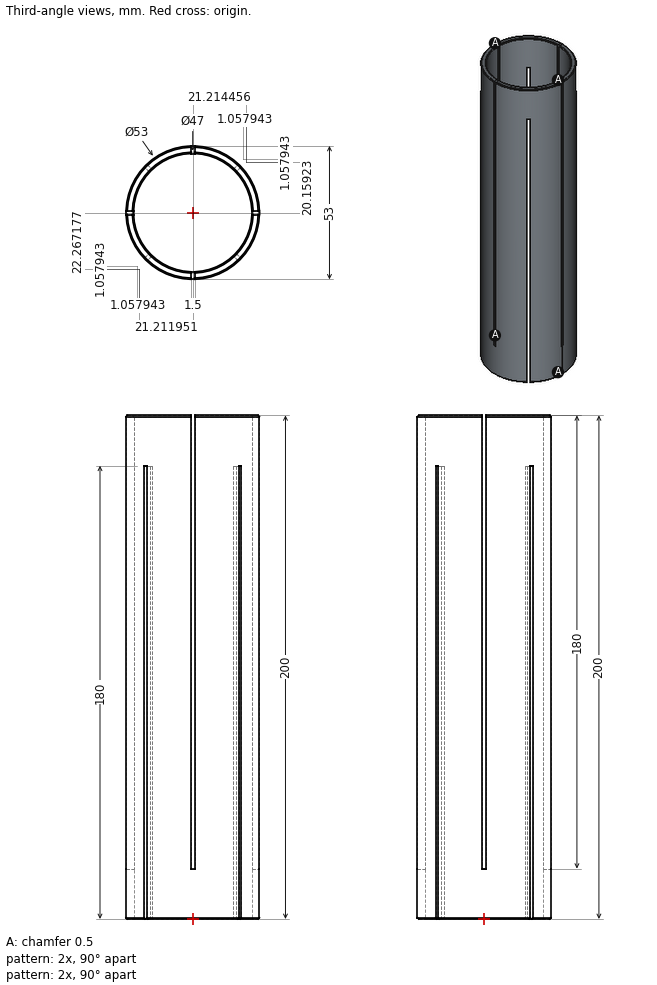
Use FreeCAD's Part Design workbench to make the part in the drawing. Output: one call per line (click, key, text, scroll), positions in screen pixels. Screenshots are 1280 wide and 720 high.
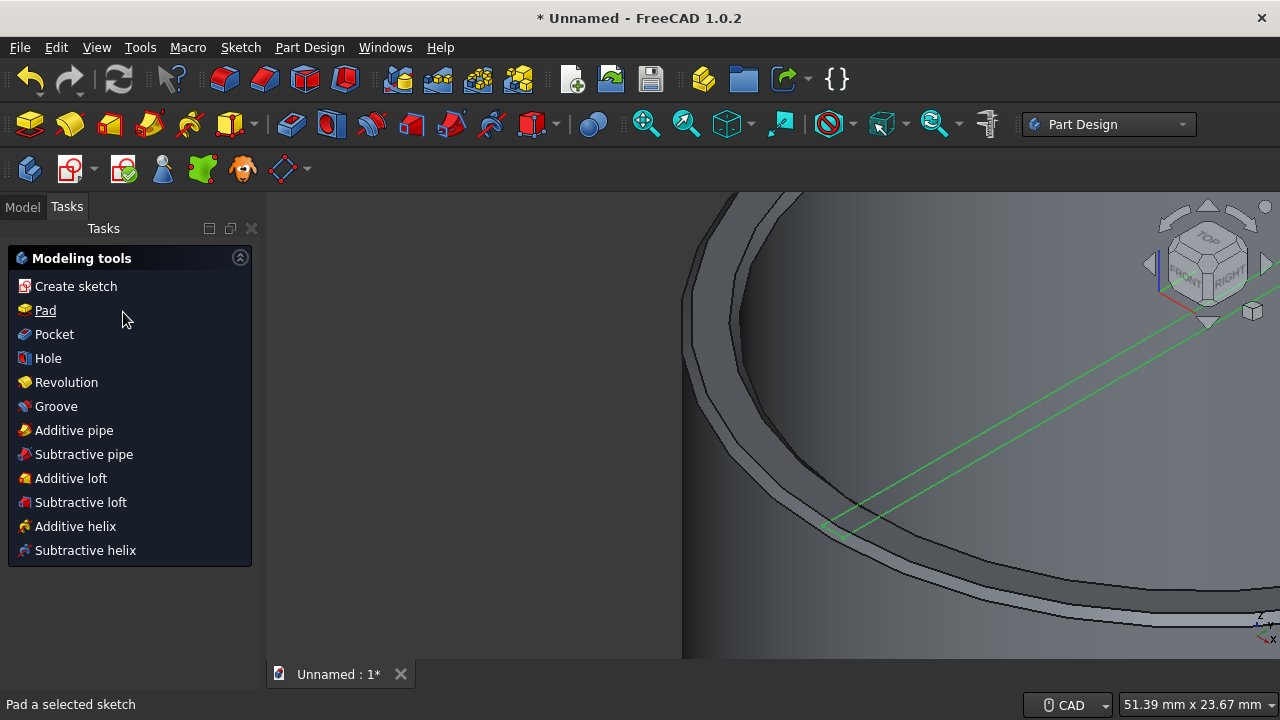
click(292, 124)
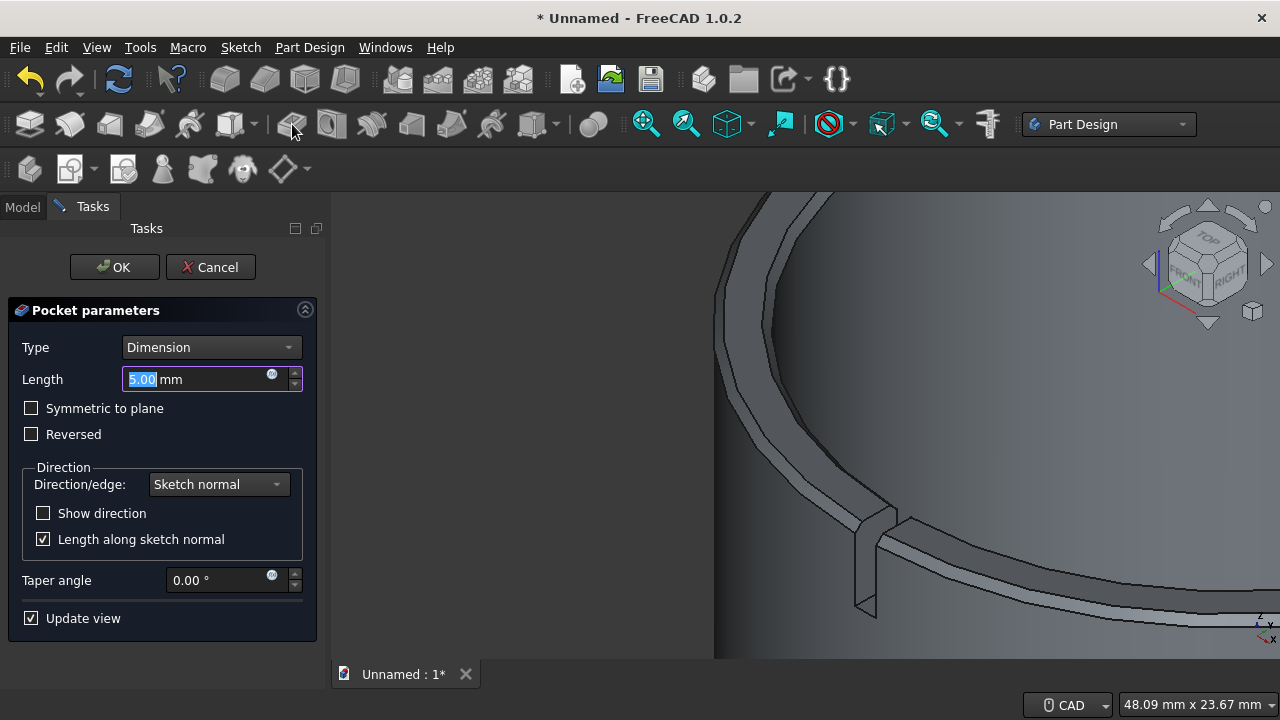
text(180)
key(Tab)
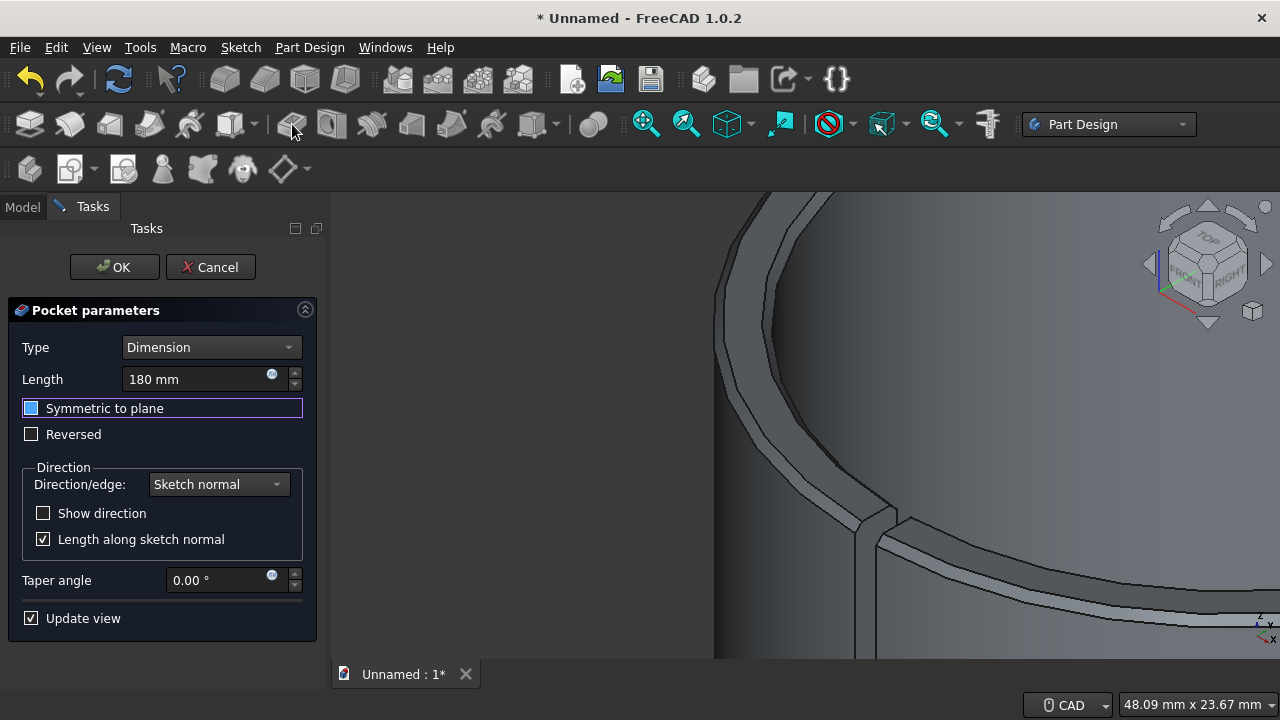
click(115, 267)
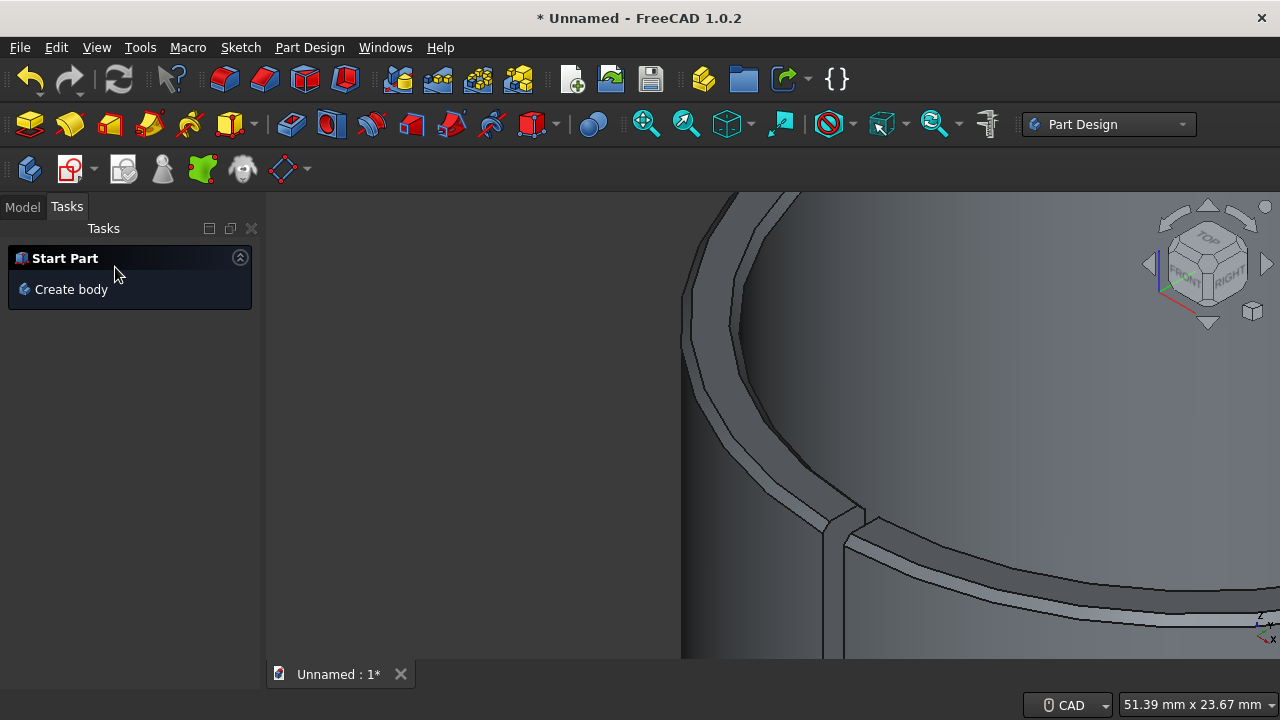
click(648, 124)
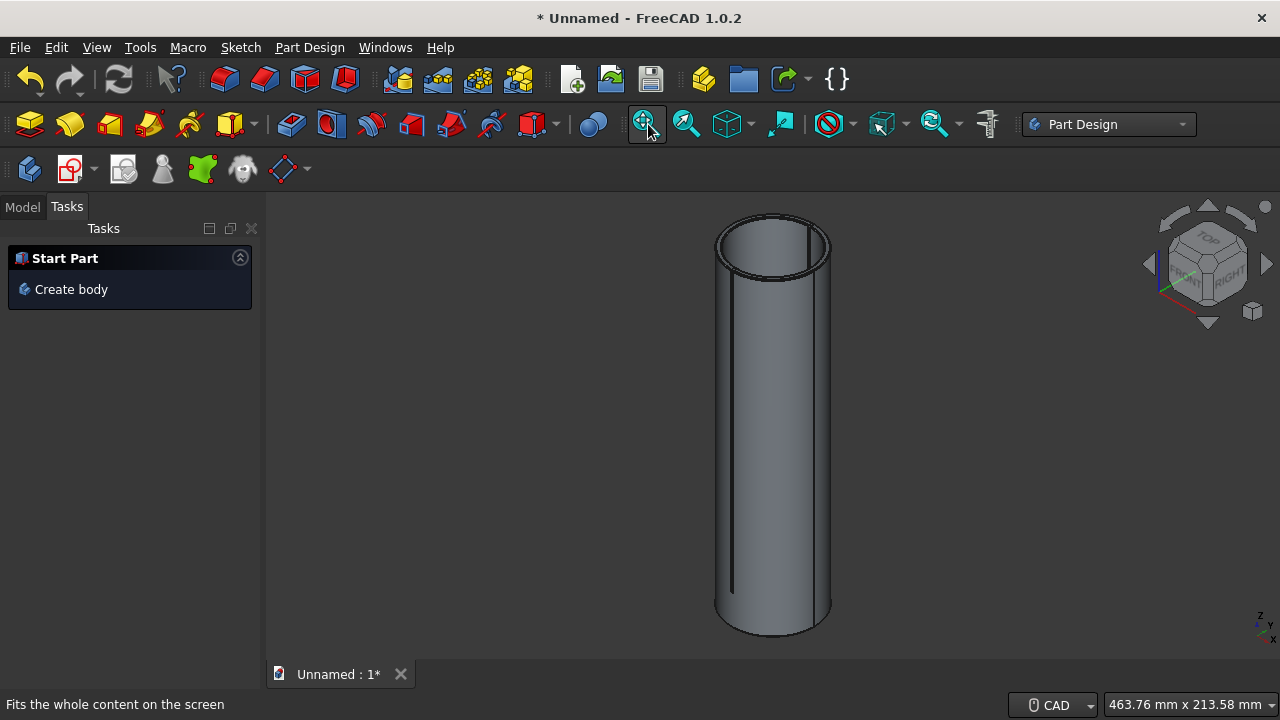
click(23, 206)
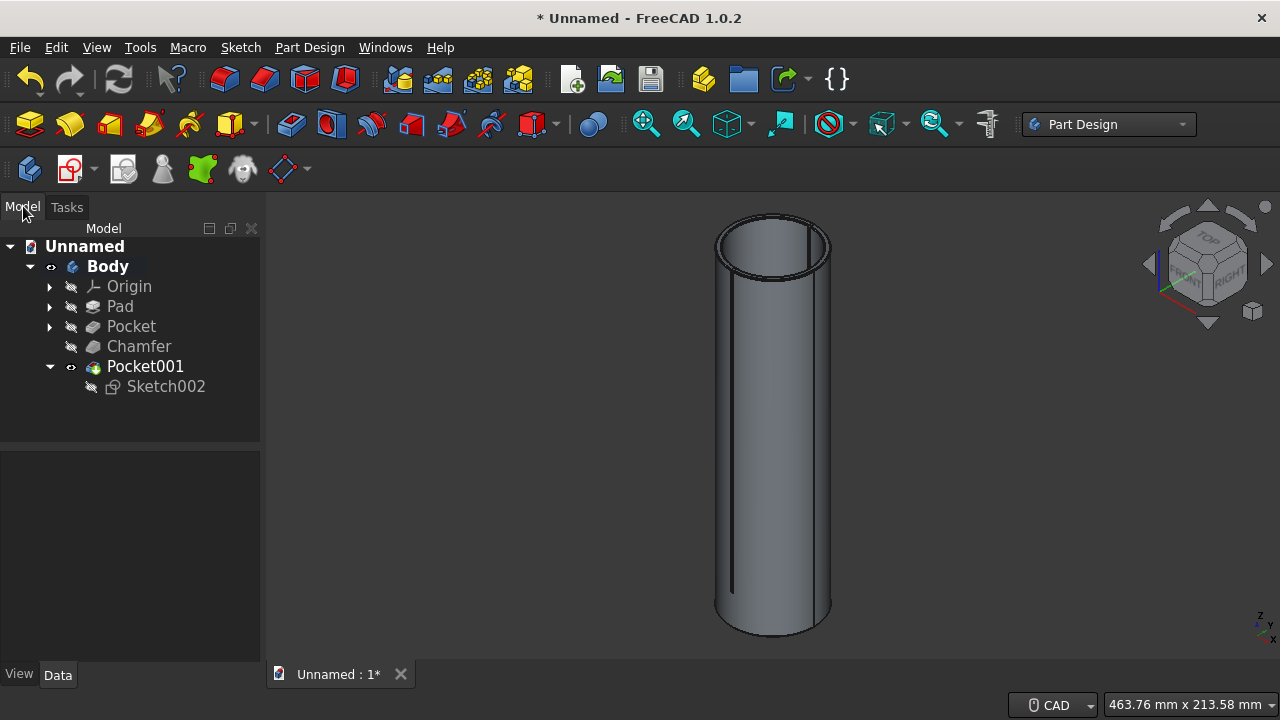
click(116, 367)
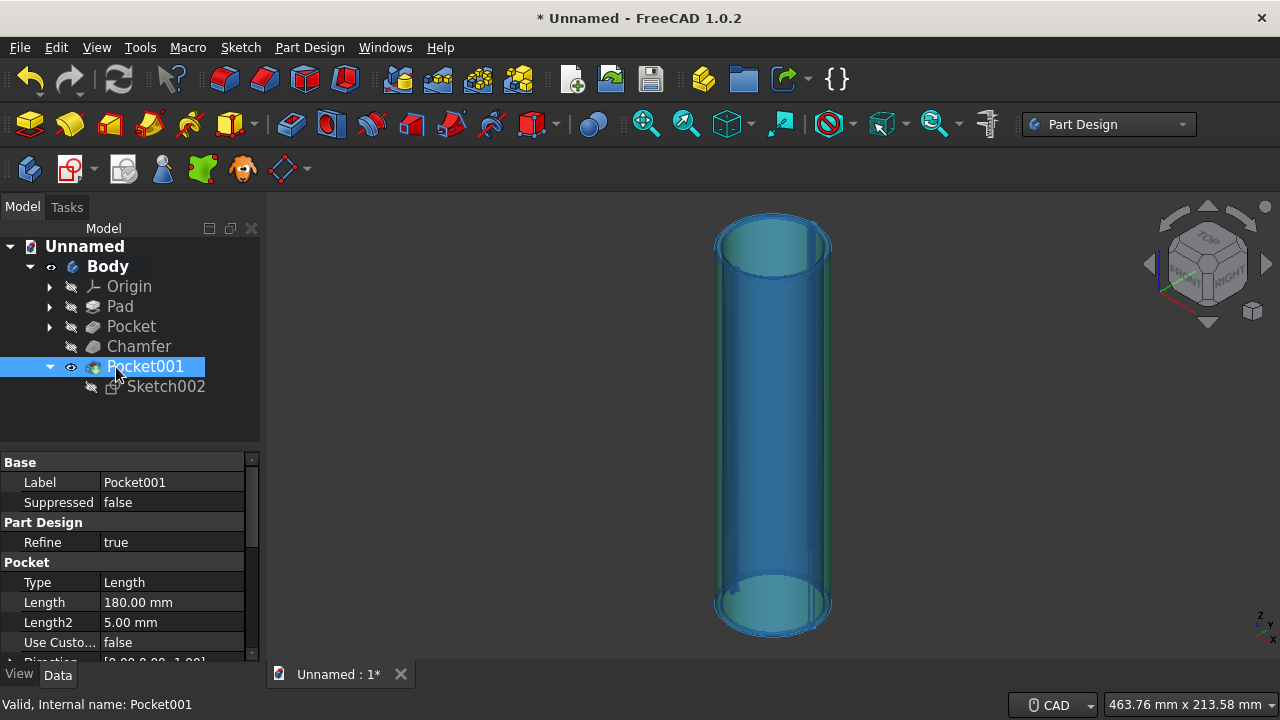
click(478, 80)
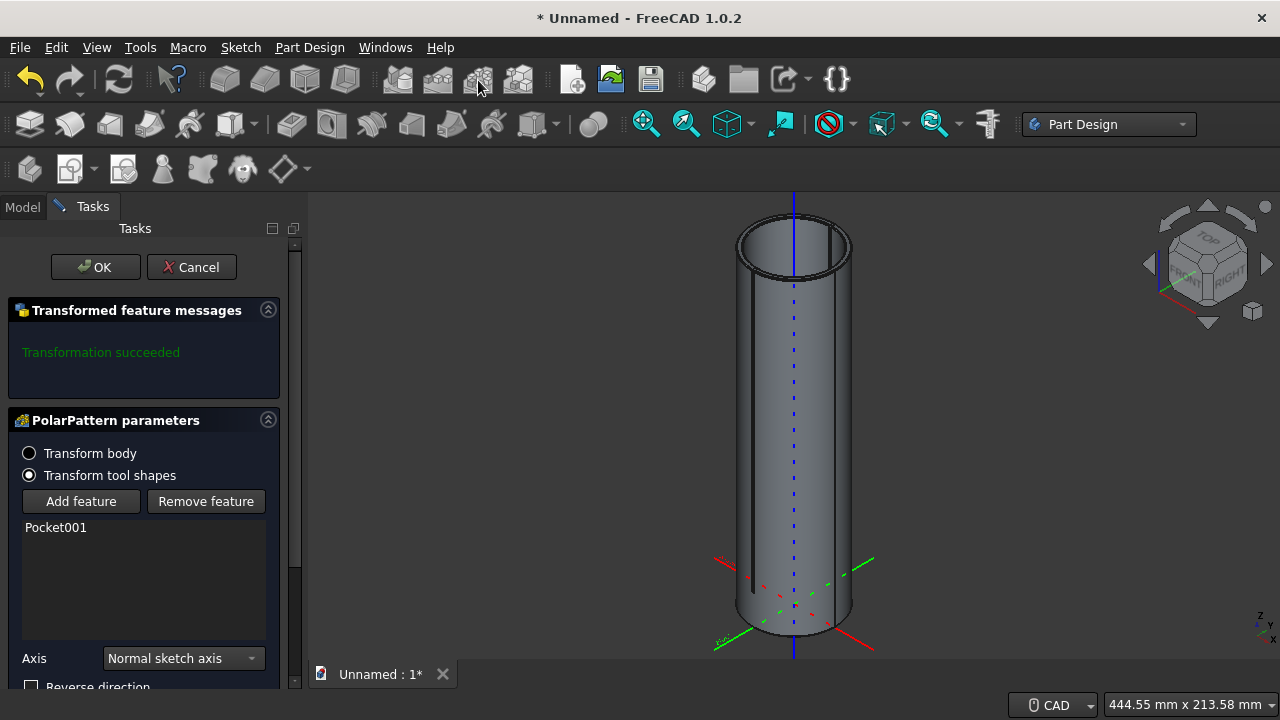
click(184, 658)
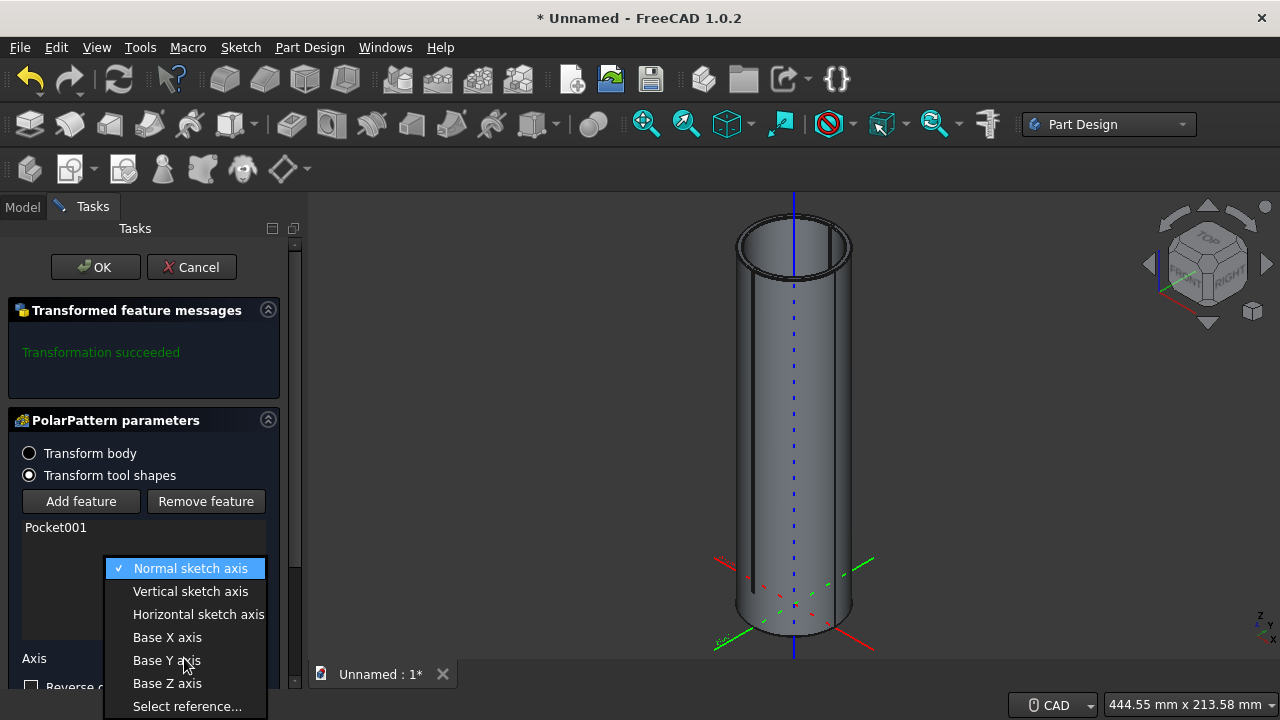
click(184, 684)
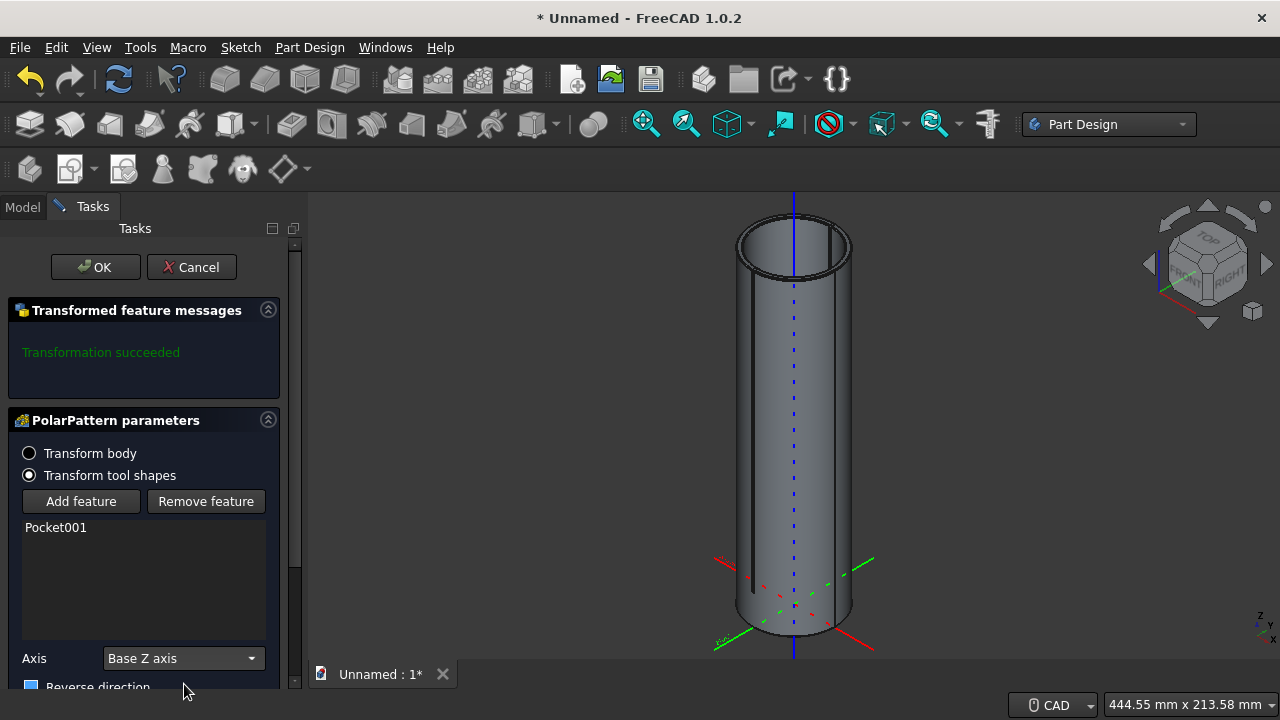
scroll(295, 463, down, 2)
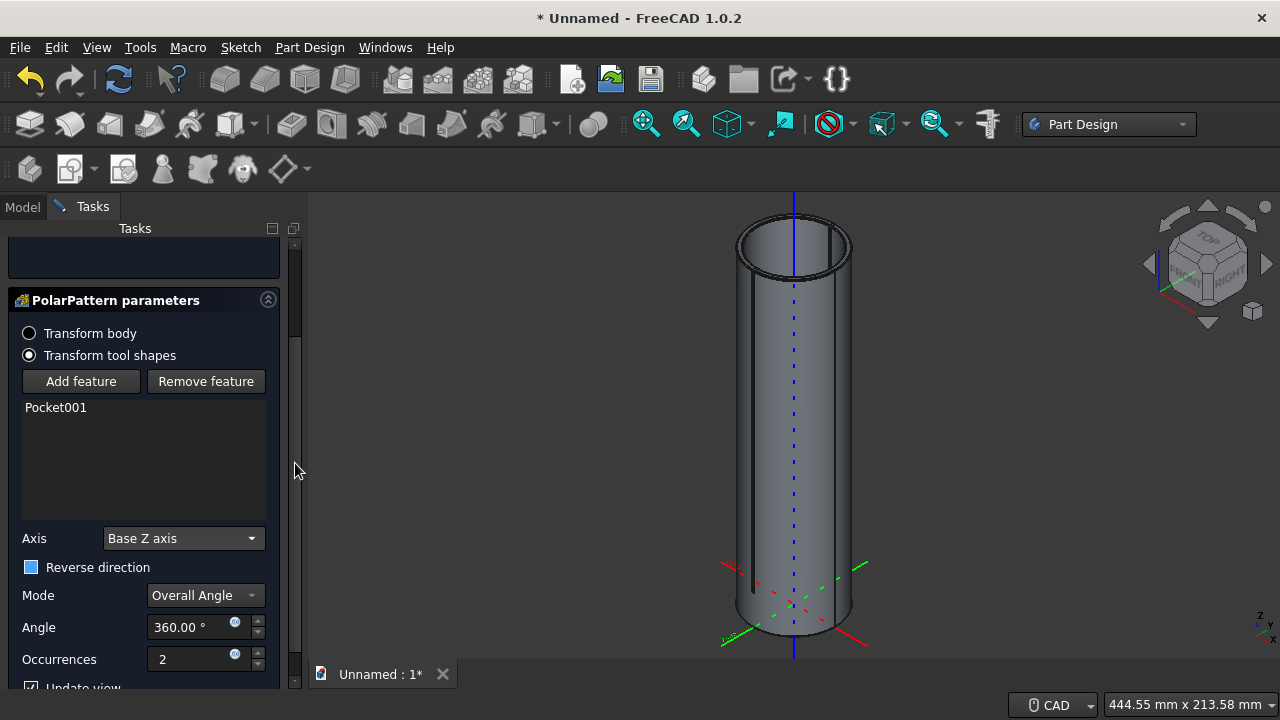
click(206, 596)